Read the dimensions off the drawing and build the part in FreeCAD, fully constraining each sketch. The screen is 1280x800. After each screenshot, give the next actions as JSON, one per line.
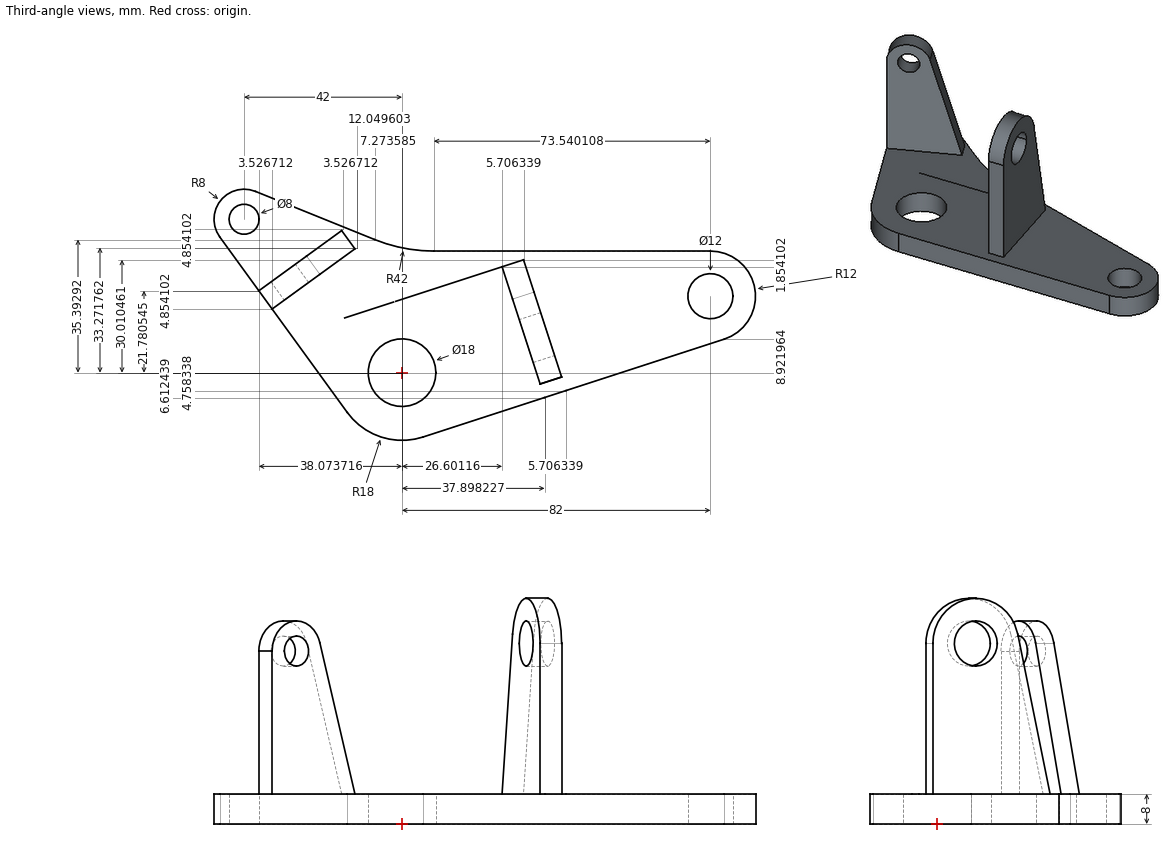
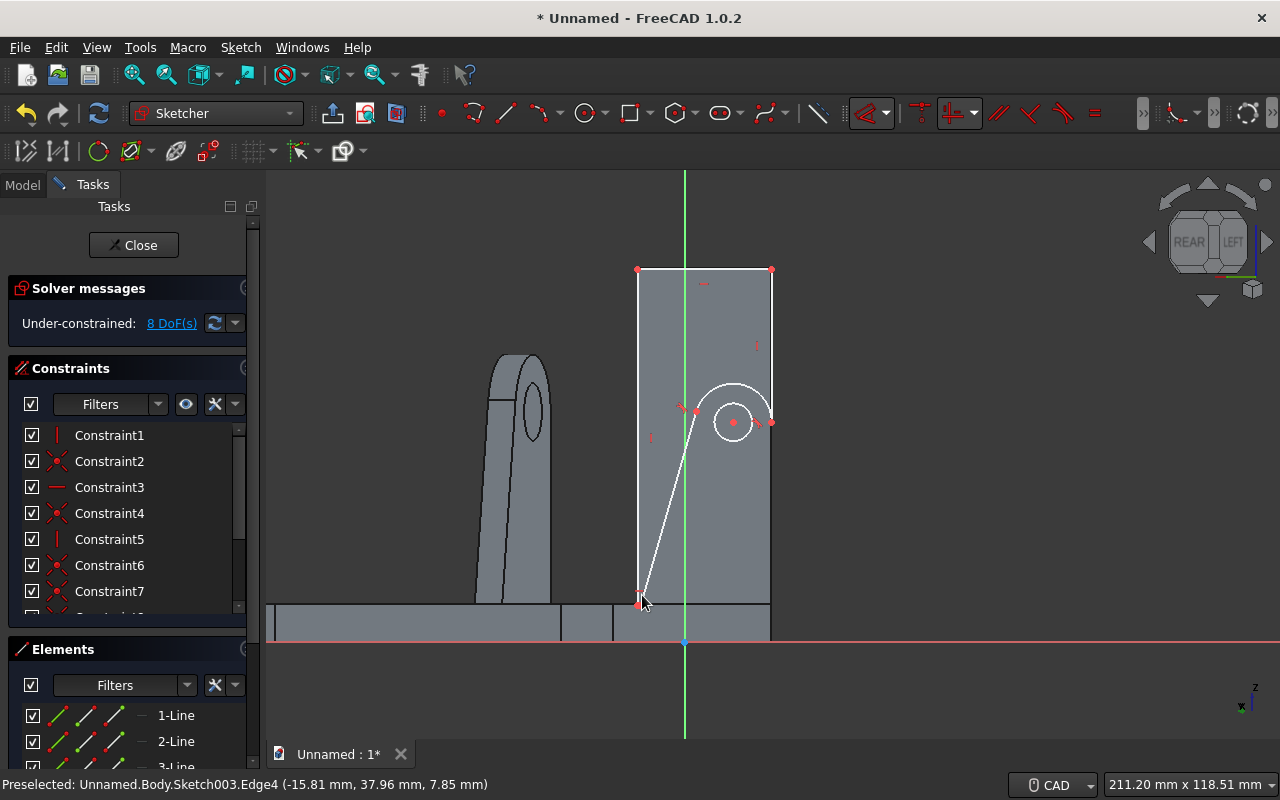
{"action": "left_click", "coordinate": [758, 393]}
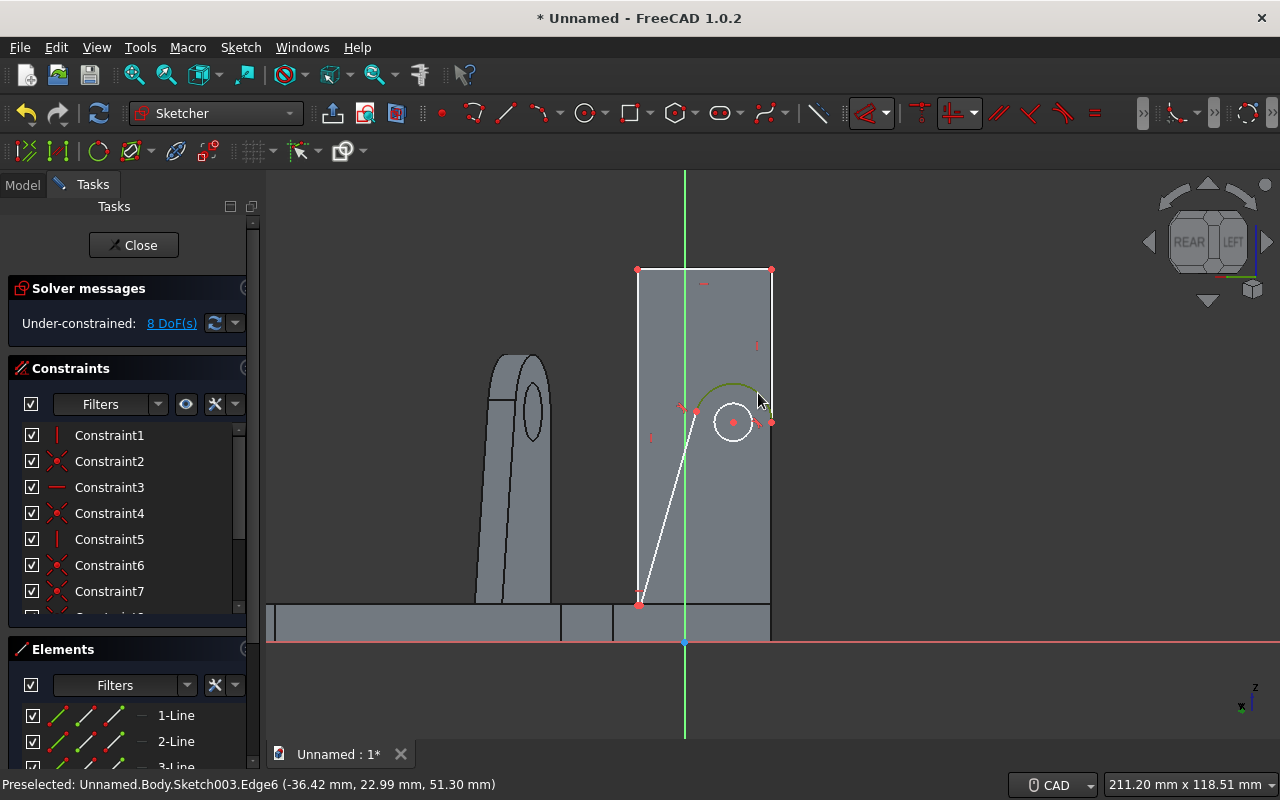
{"action": "left_click", "coordinate": [888, 114]}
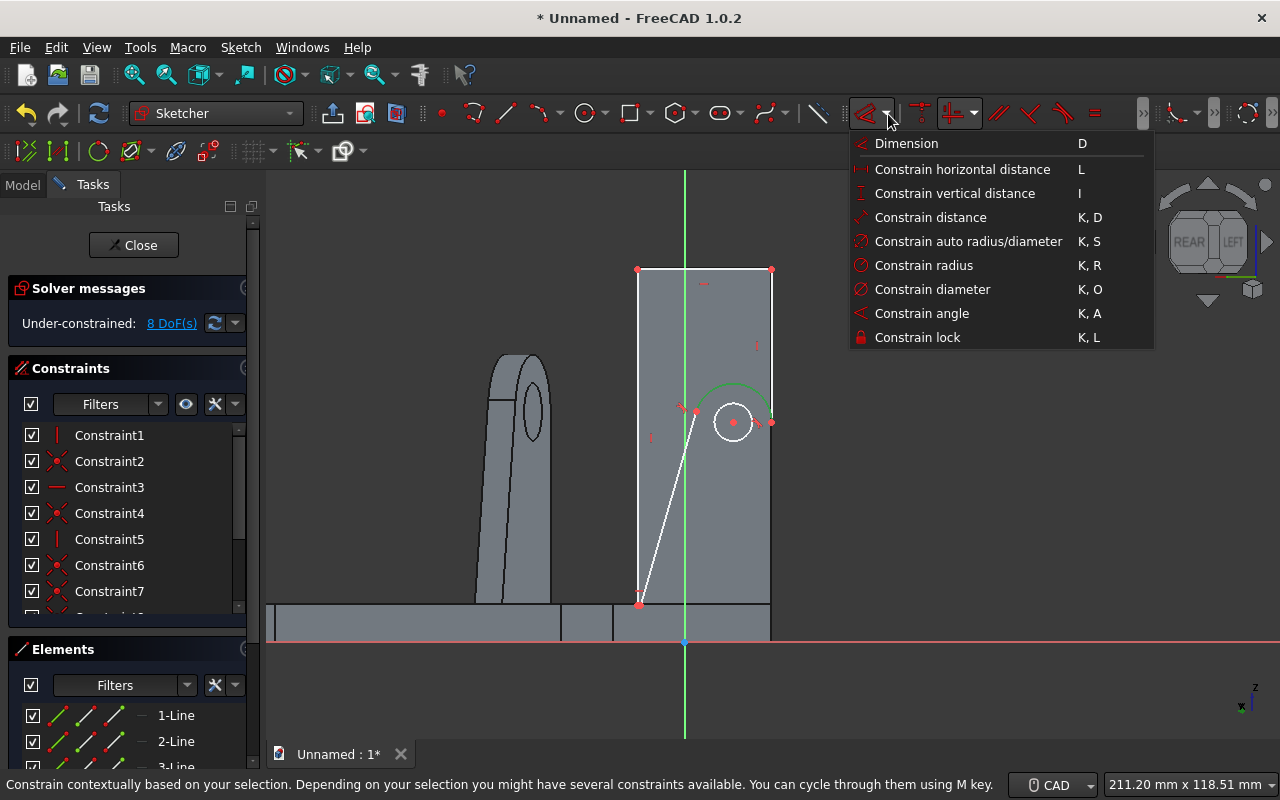
{"action": "left_click", "coordinate": [1002, 265]}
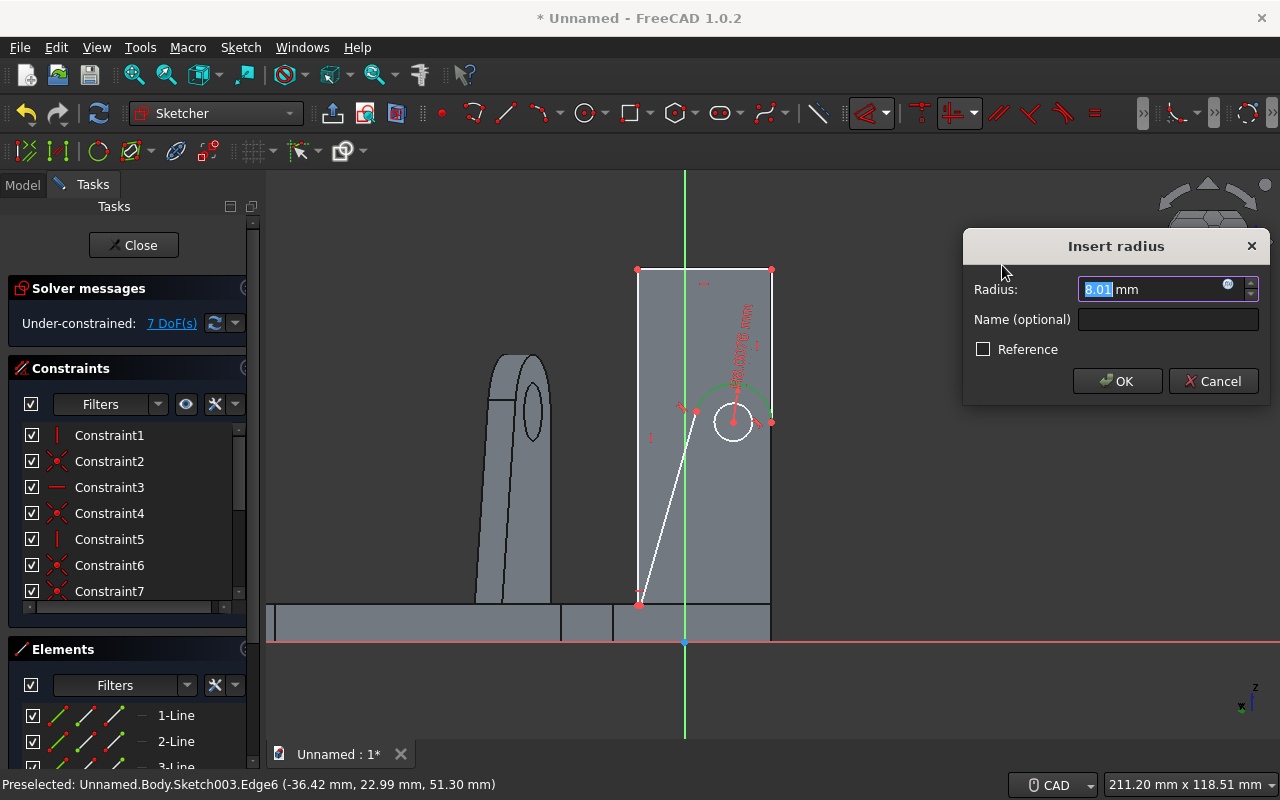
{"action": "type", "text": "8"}
{"action": "key", "text": "Return"}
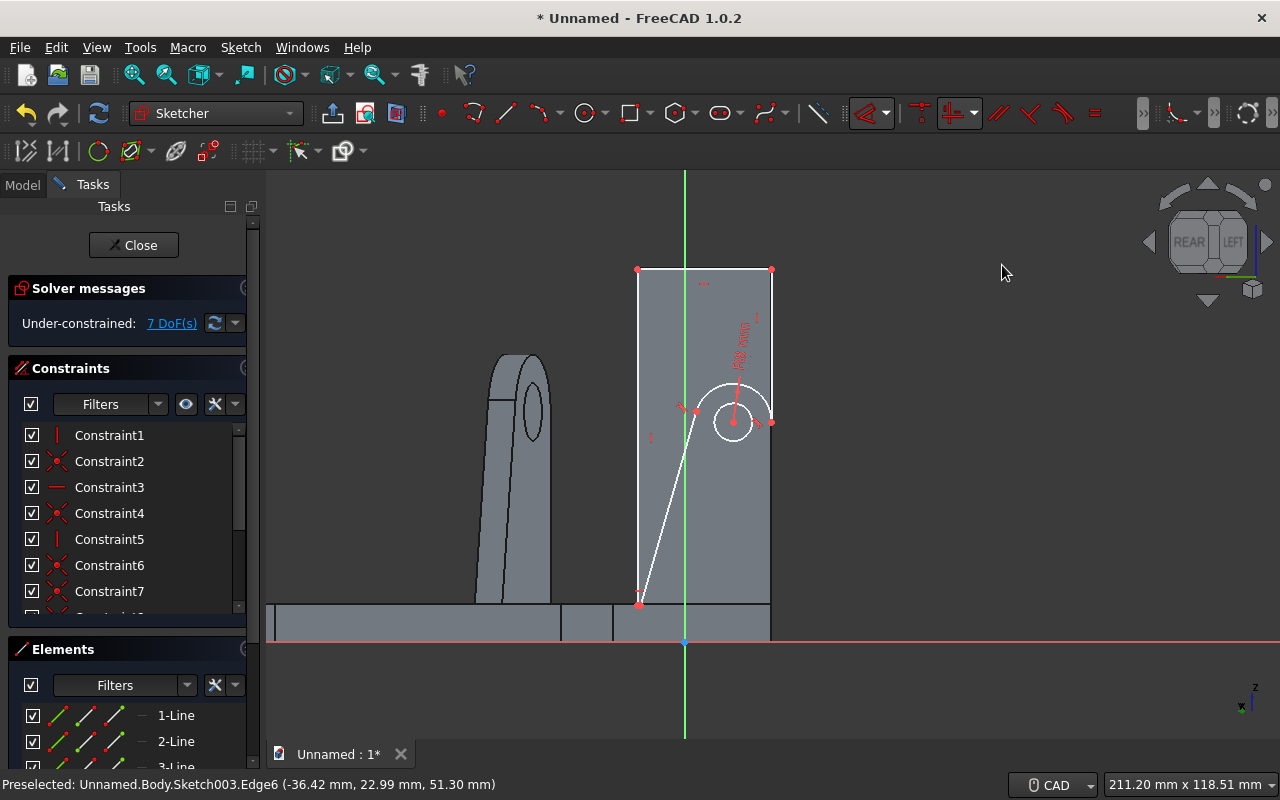
{"action": "left_click", "coordinate": [746, 409]}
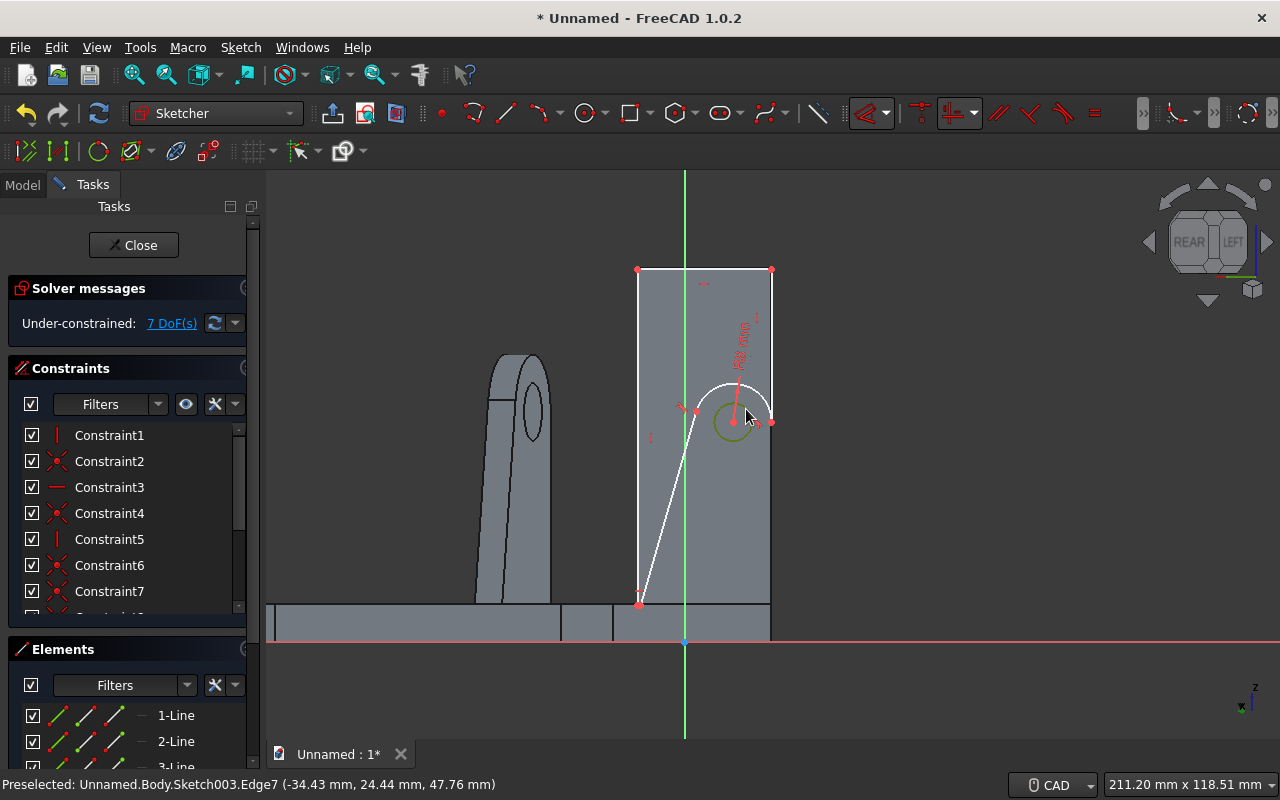
{"action": "key", "text": "k o"}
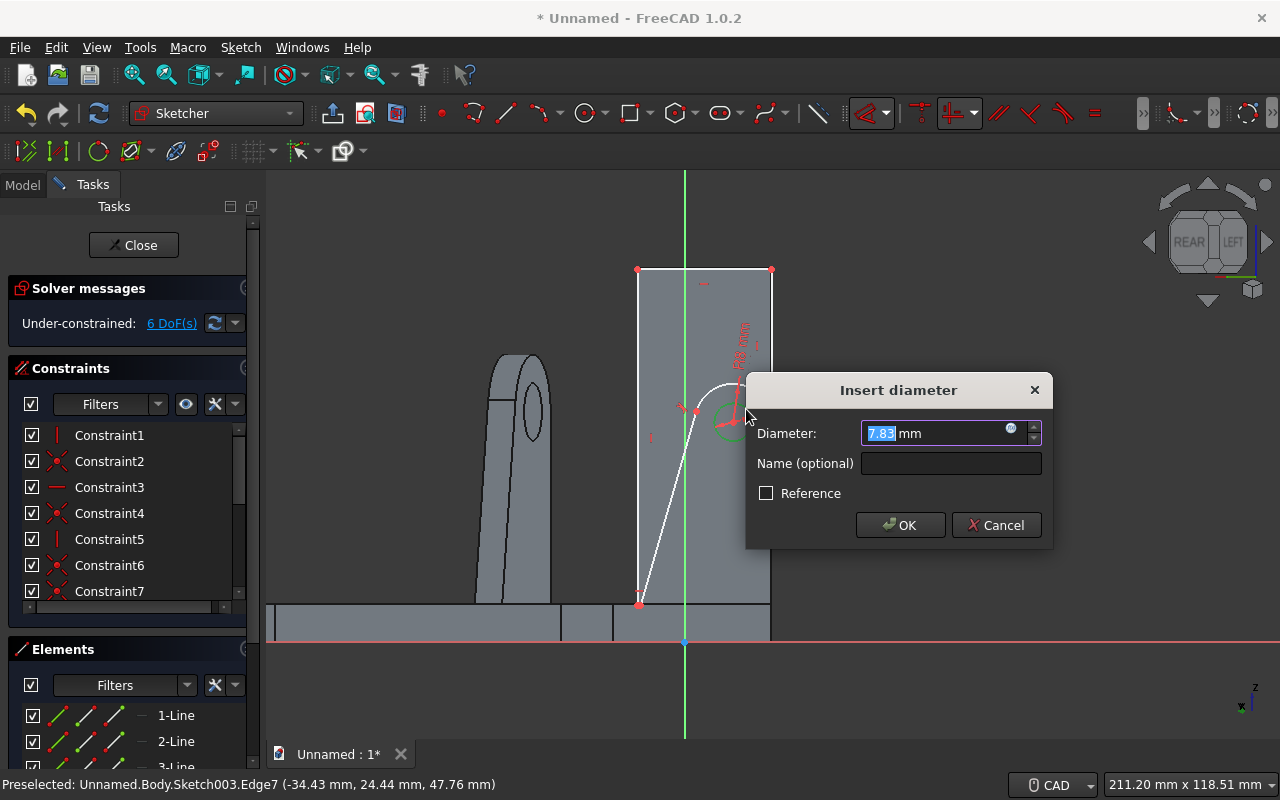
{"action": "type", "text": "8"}
{"action": "key", "text": "Return"}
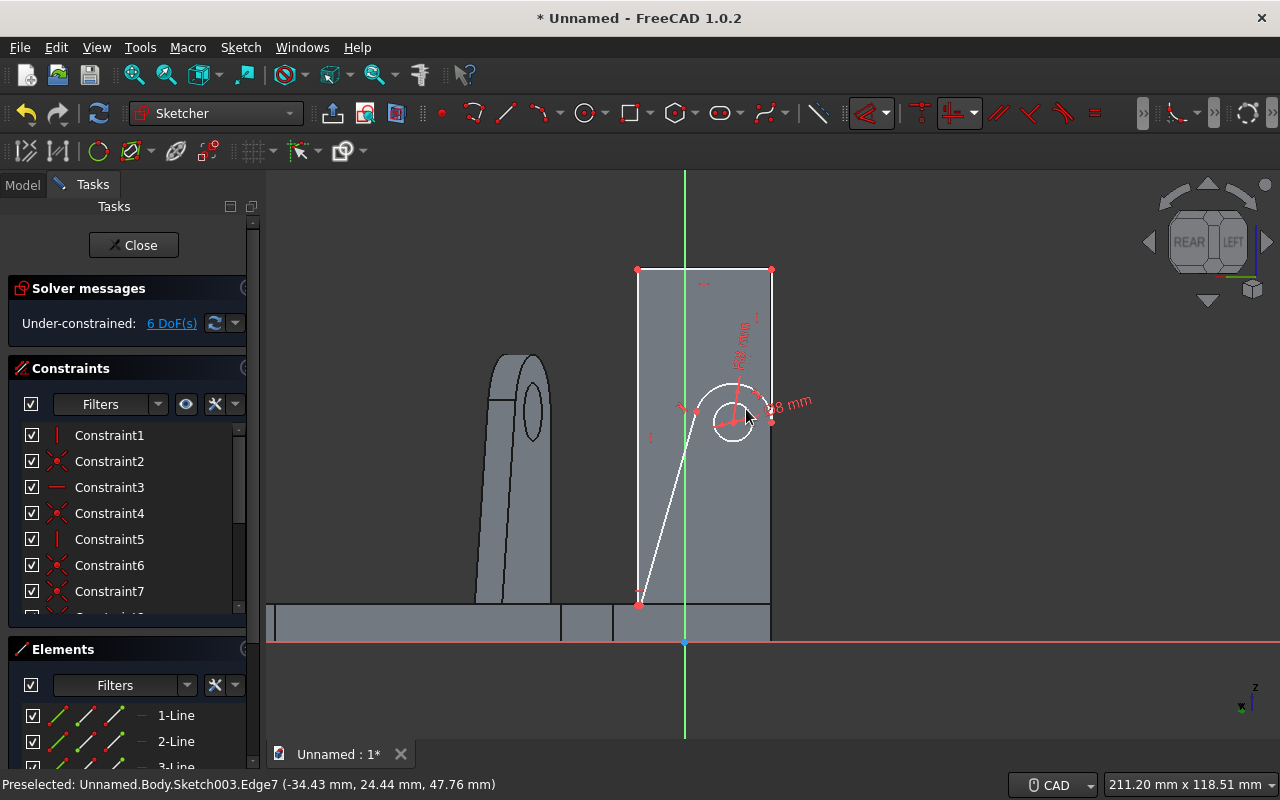
{"action": "left_click", "coordinate": [772, 376]}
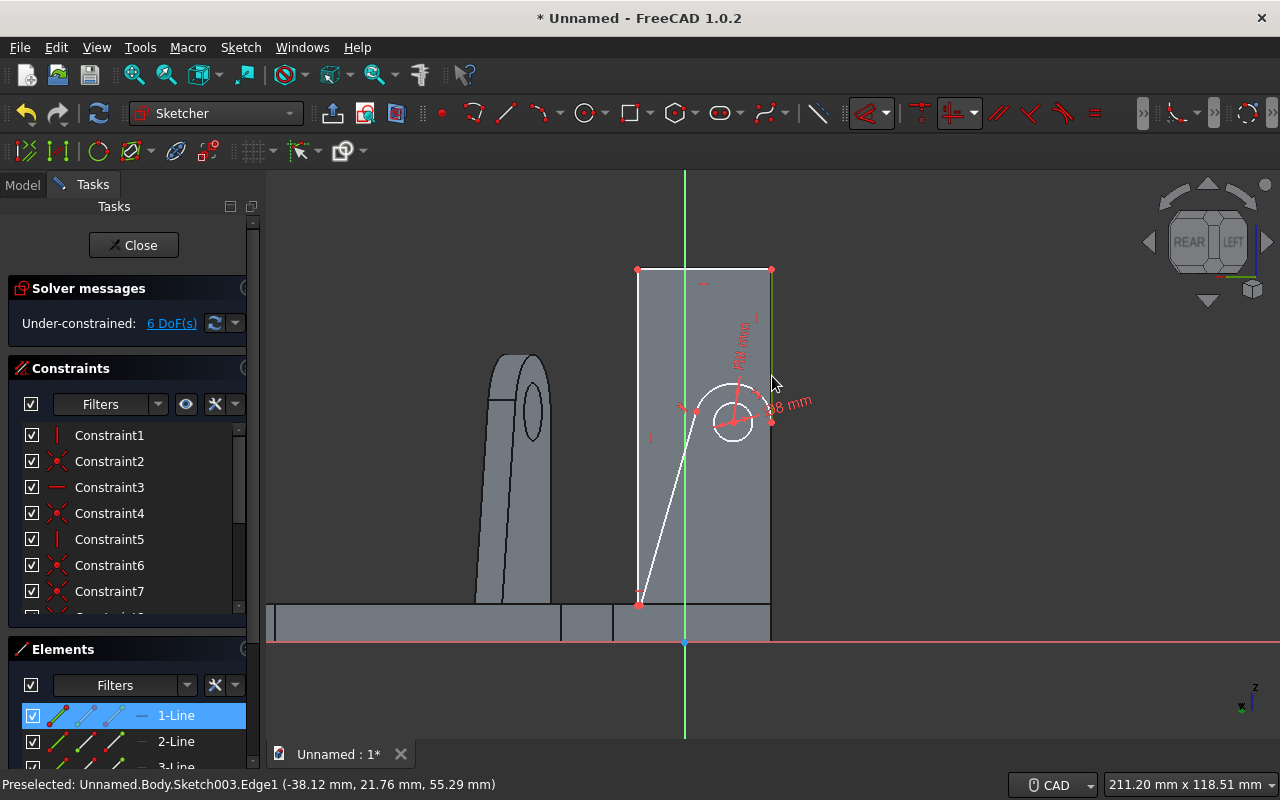
{"action": "key", "text": "i"}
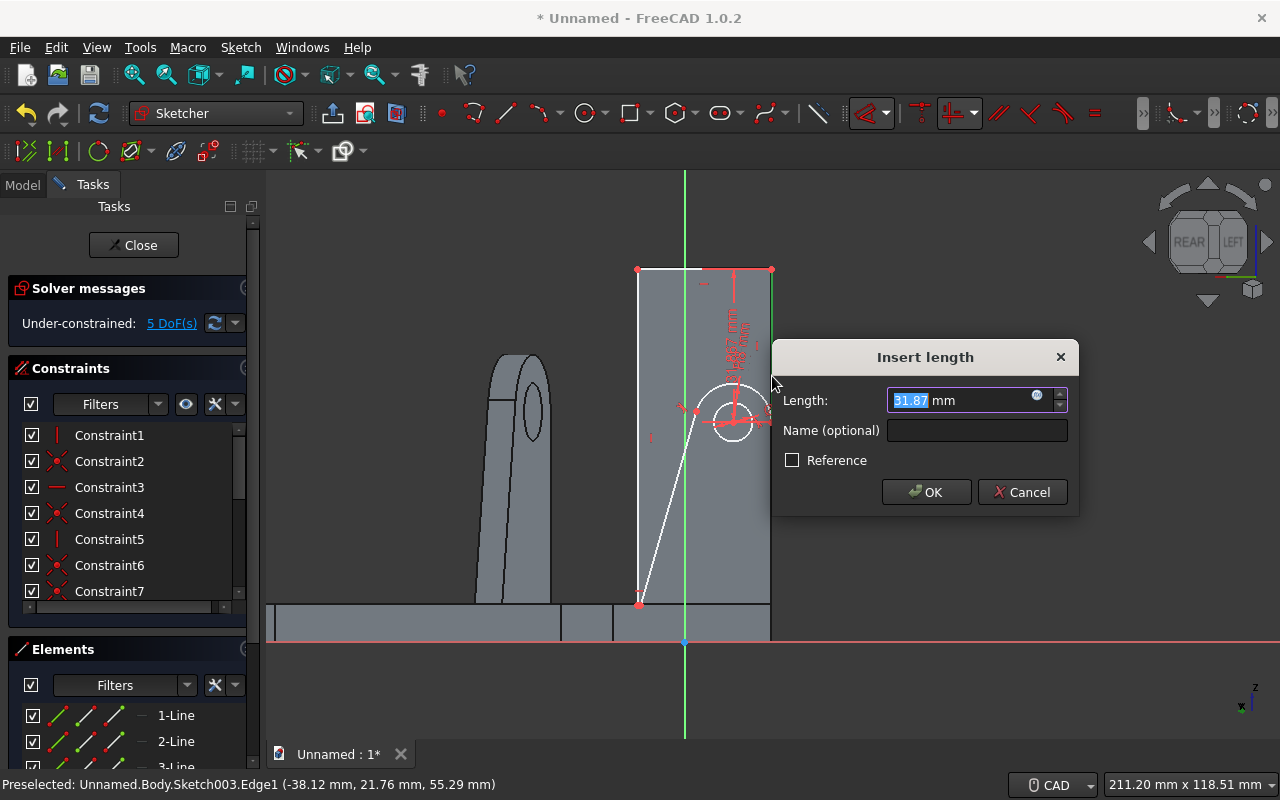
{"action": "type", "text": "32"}
{"action": "key", "text": "Return"}